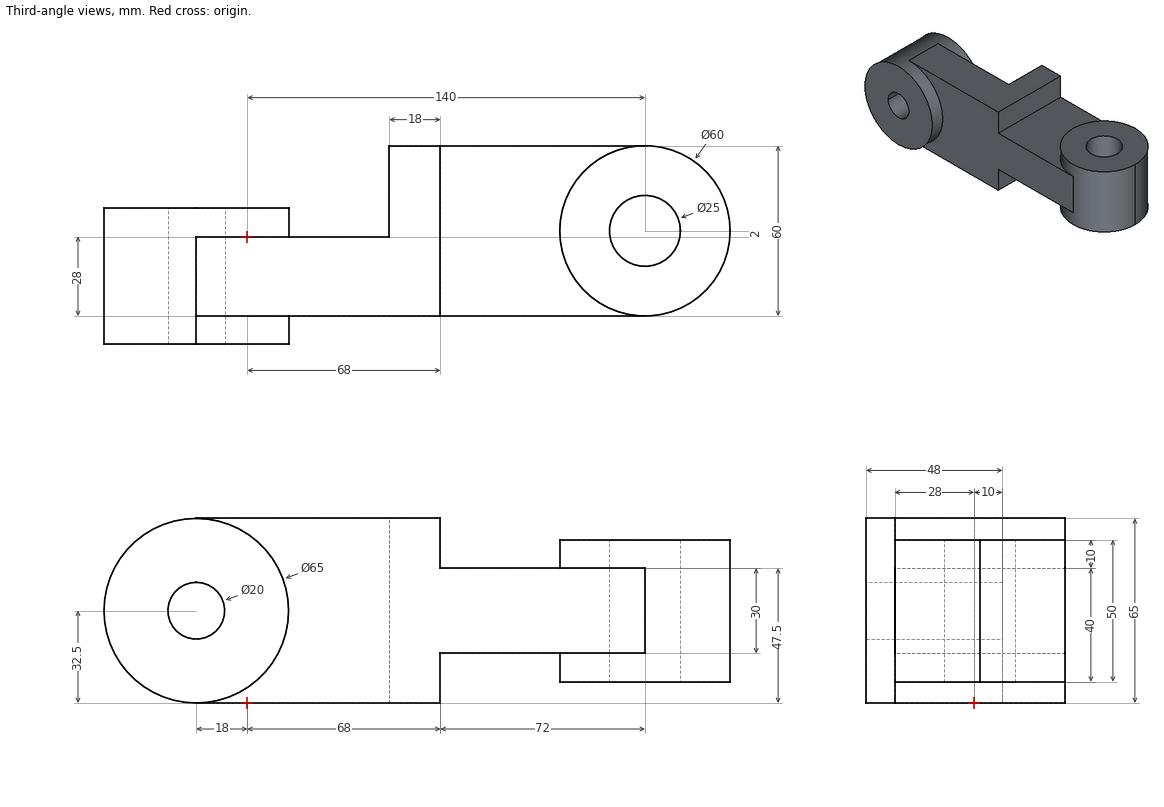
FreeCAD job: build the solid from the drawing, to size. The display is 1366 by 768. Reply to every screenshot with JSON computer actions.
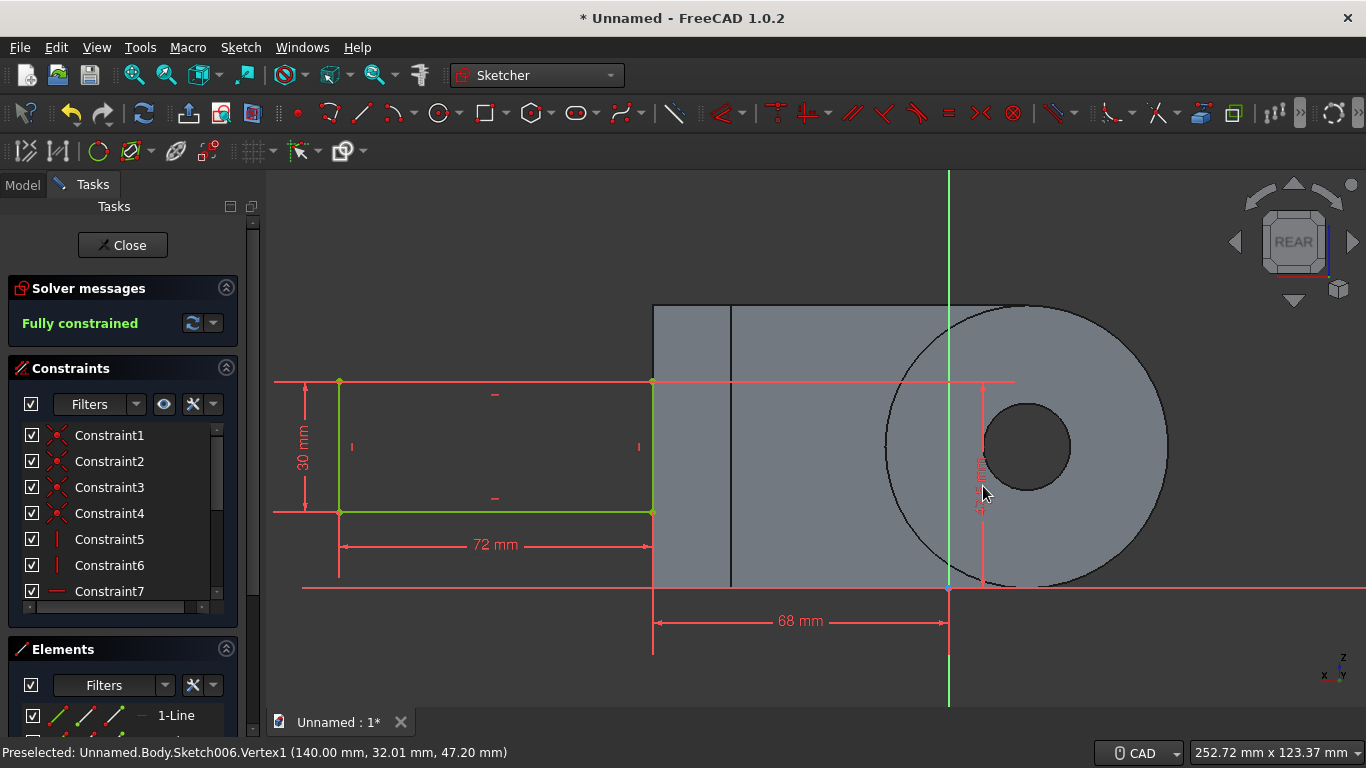
{"action": "left_click", "coordinate": [123, 245]}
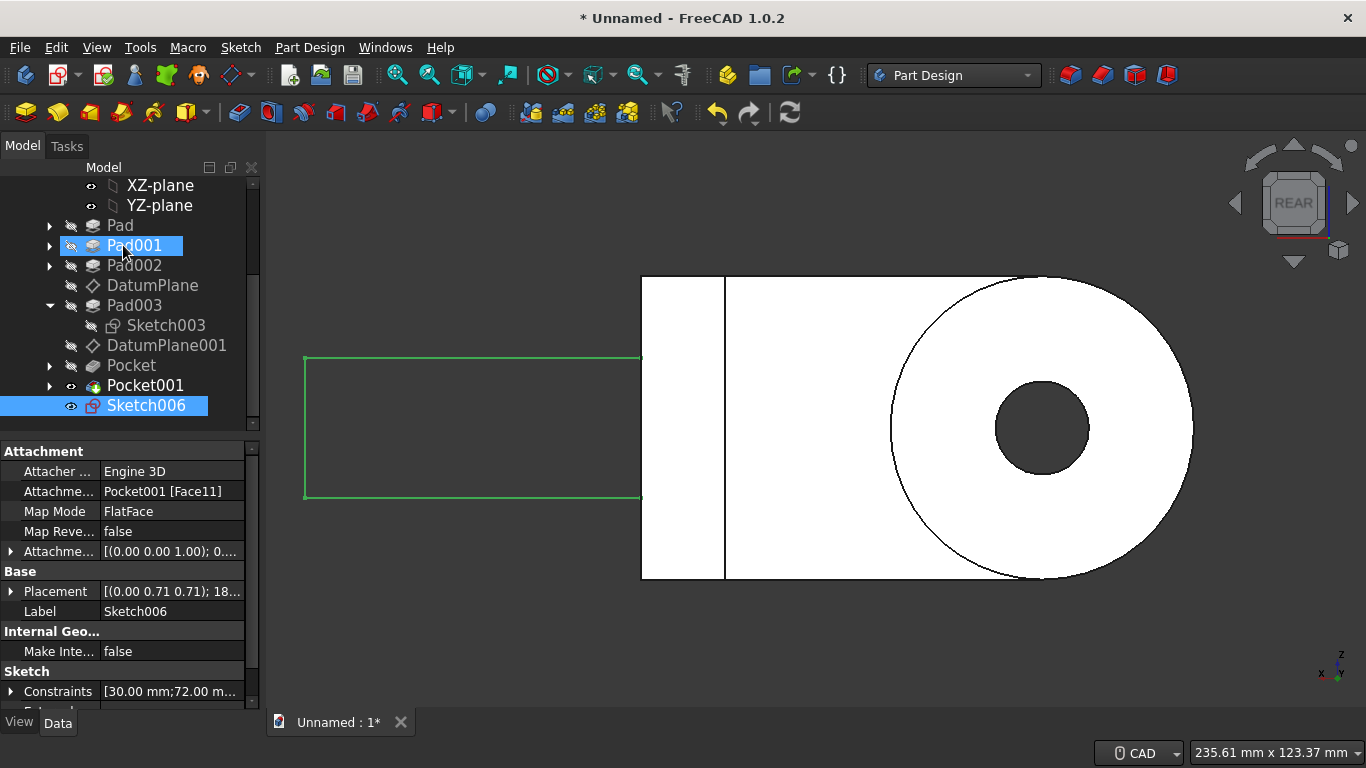
{"action": "left_click", "coordinate": [26, 112]}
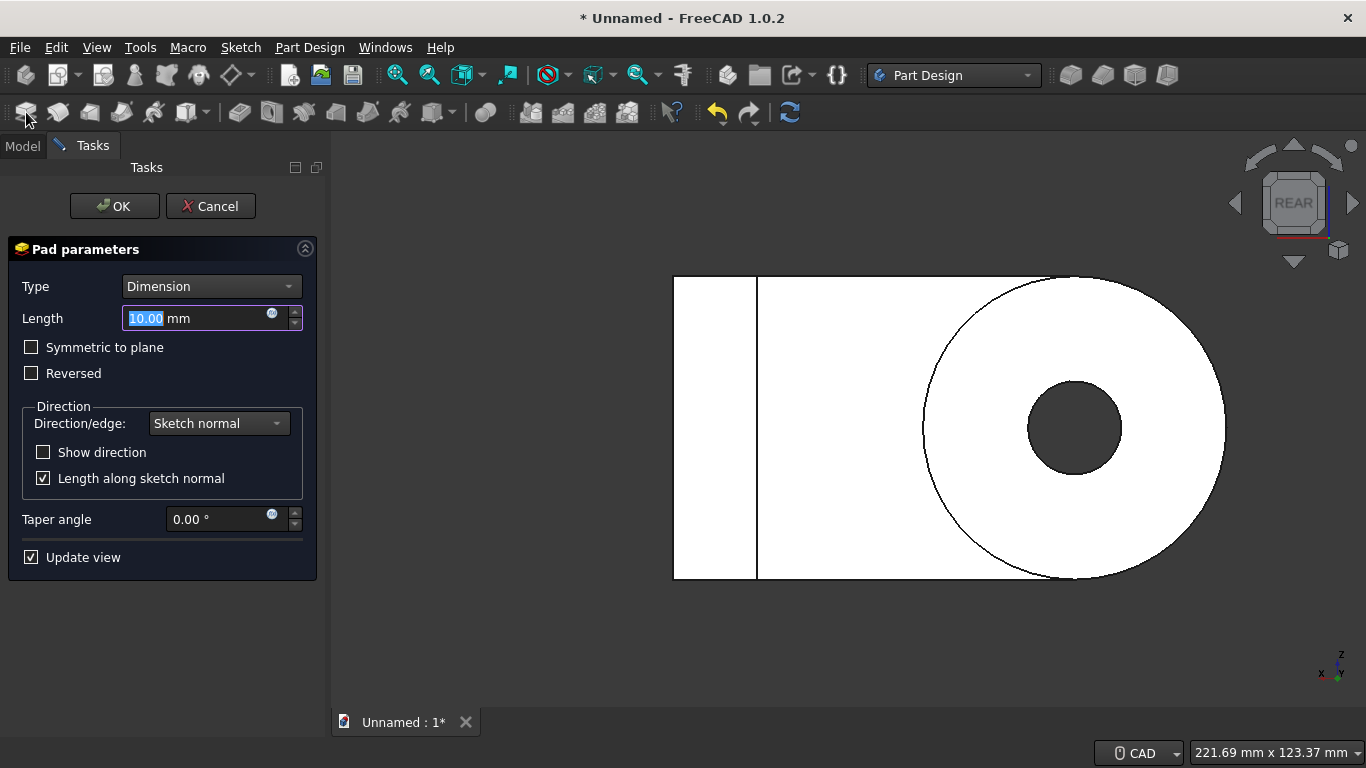
{"action": "type", "text": "60"}
{"action": "key", "text": "Tab"}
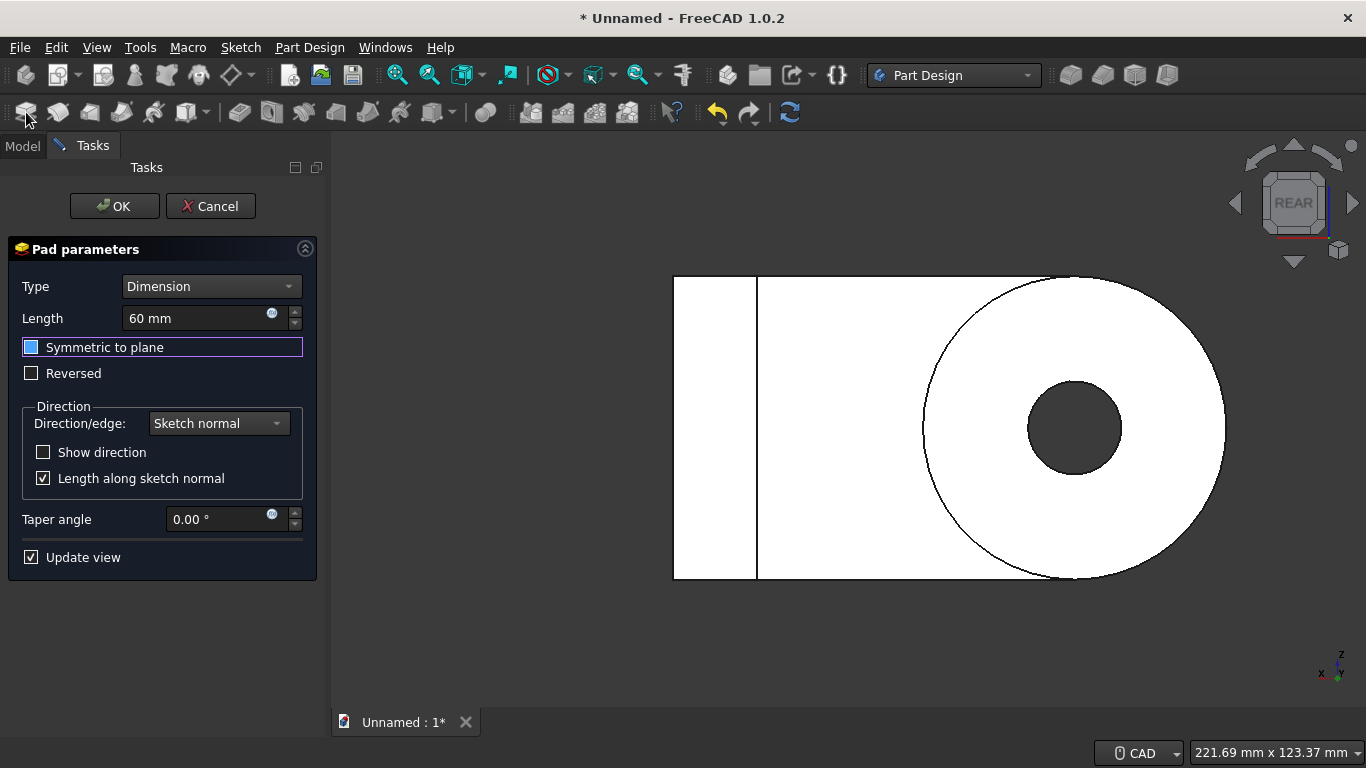
{"action": "left_click", "coordinate": [30, 373]}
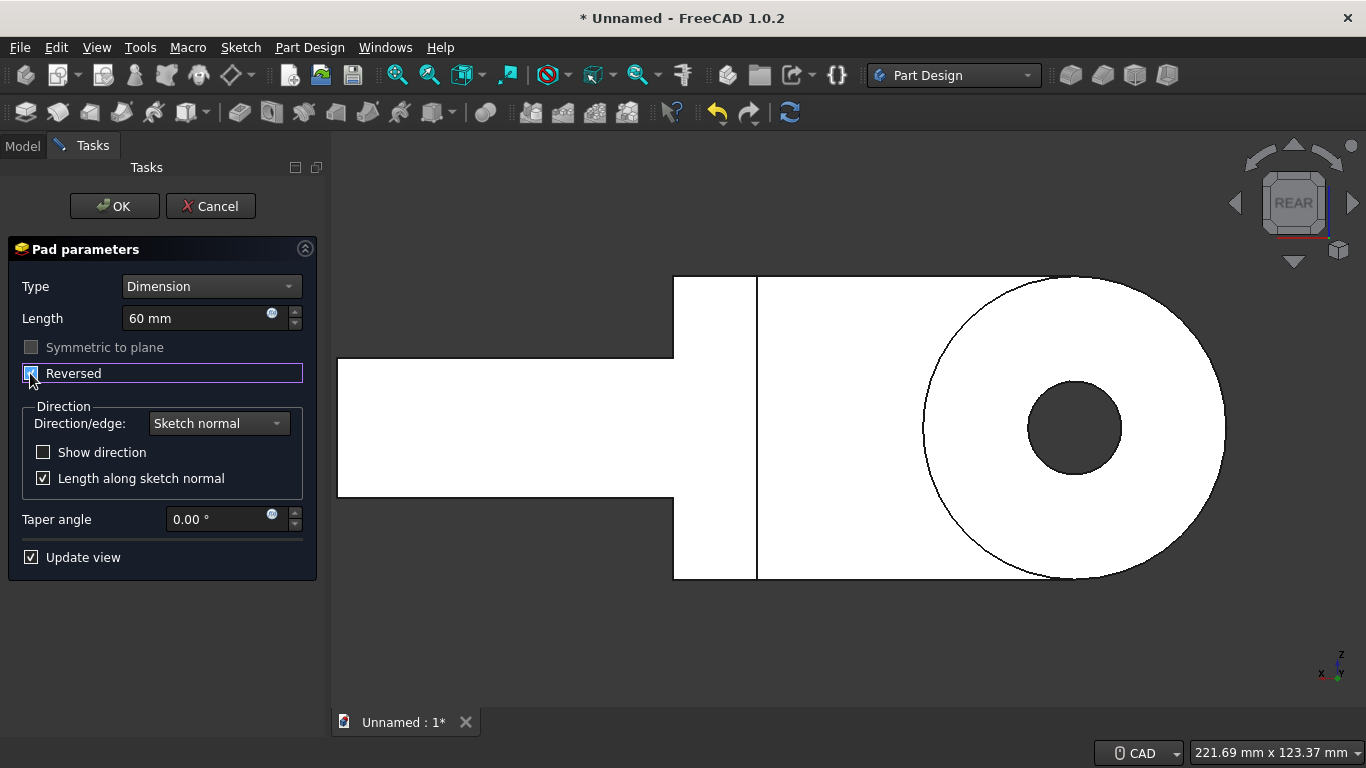
{"action": "left_click", "coordinate": [115, 206]}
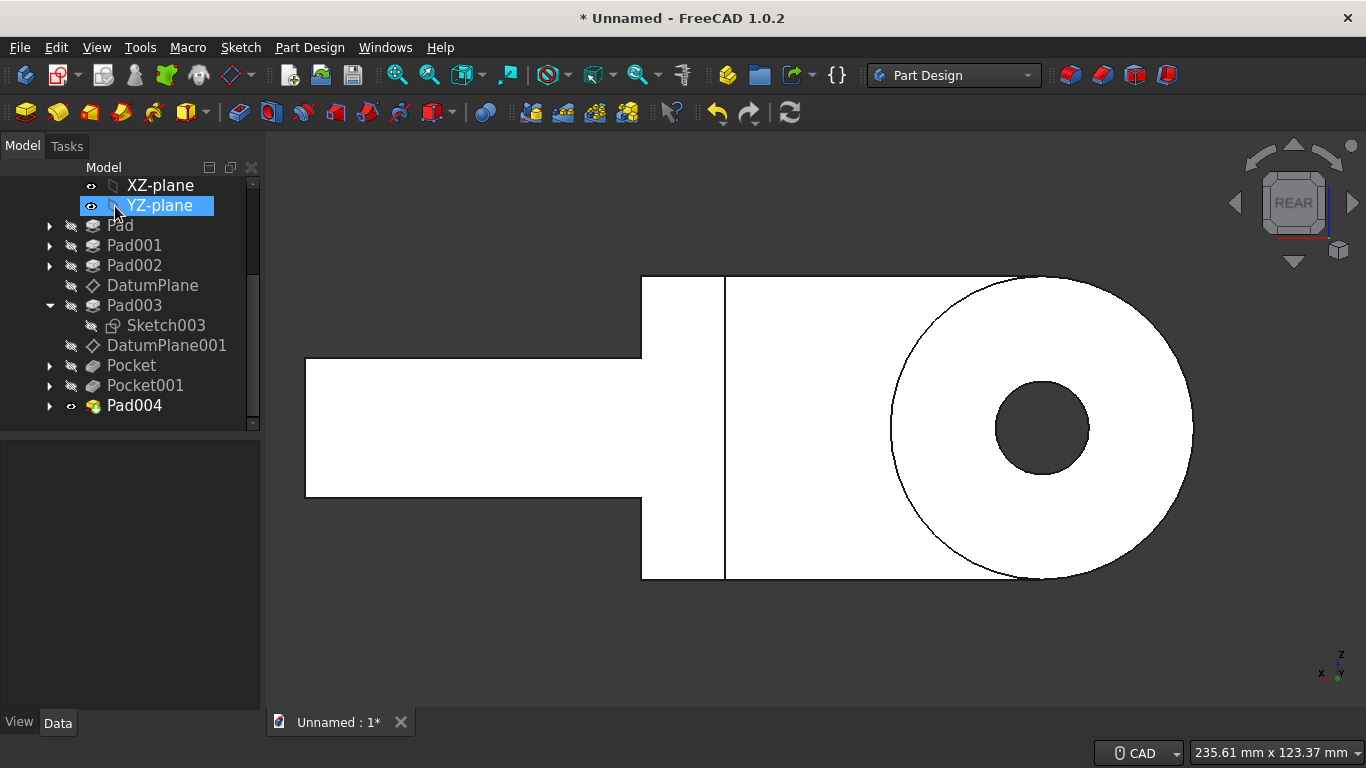
{"action": "key", "text": "0"}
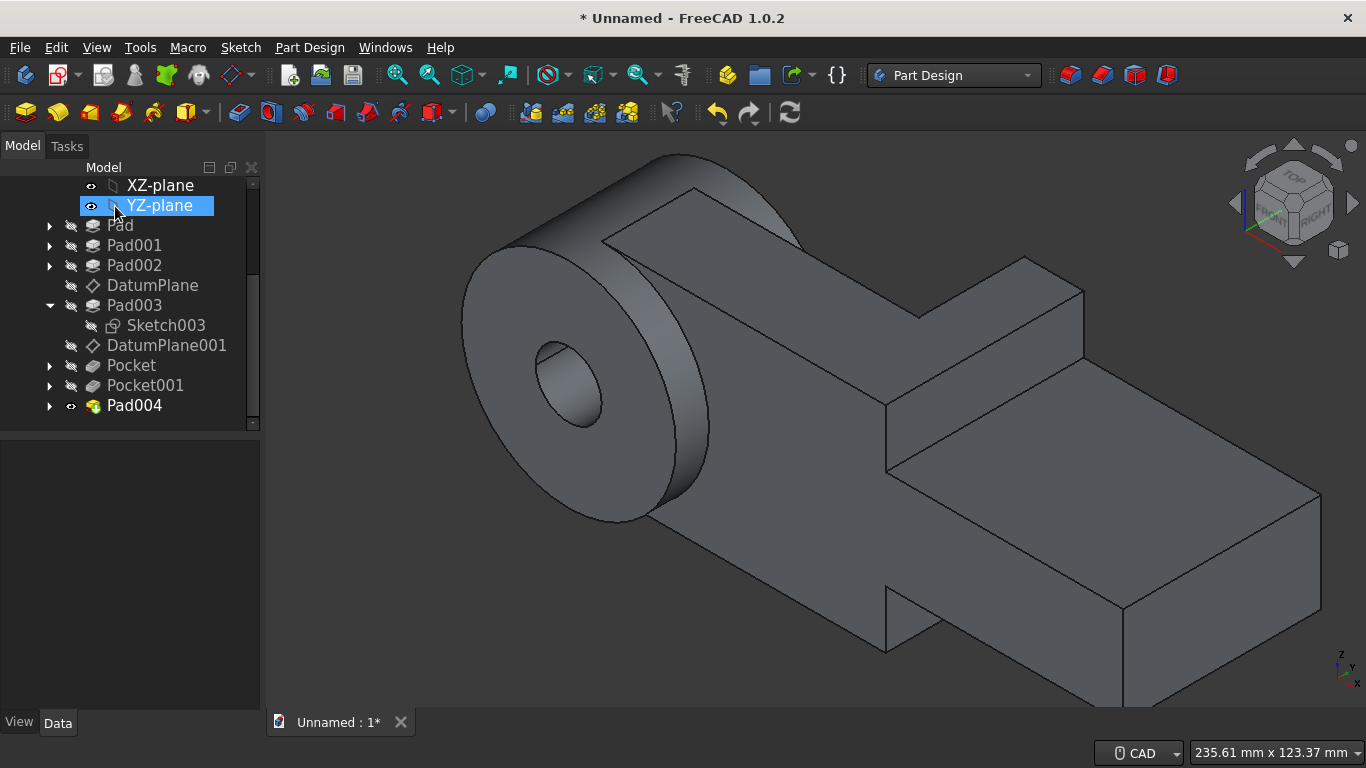
{"action": "left_click", "coordinate": [398, 76]}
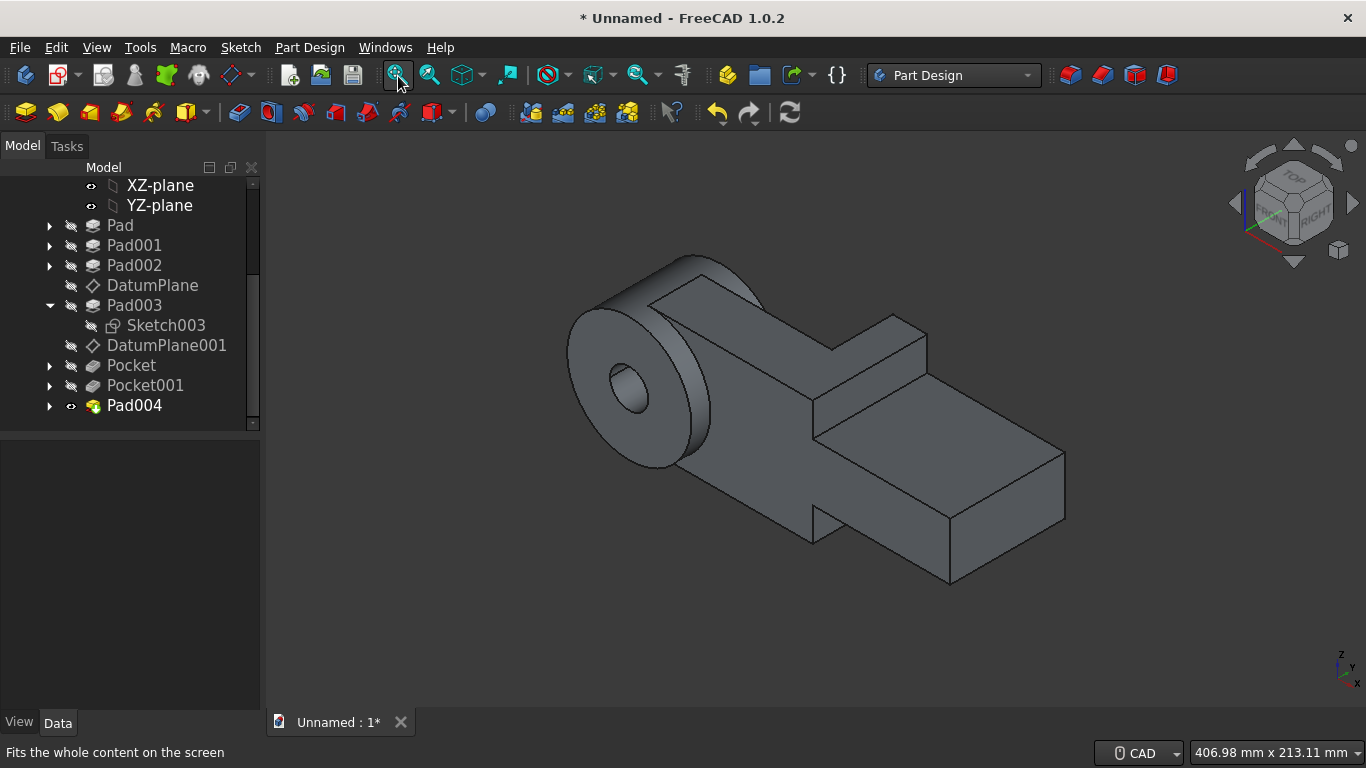
{"action": "left_click", "coordinate": [939, 445]}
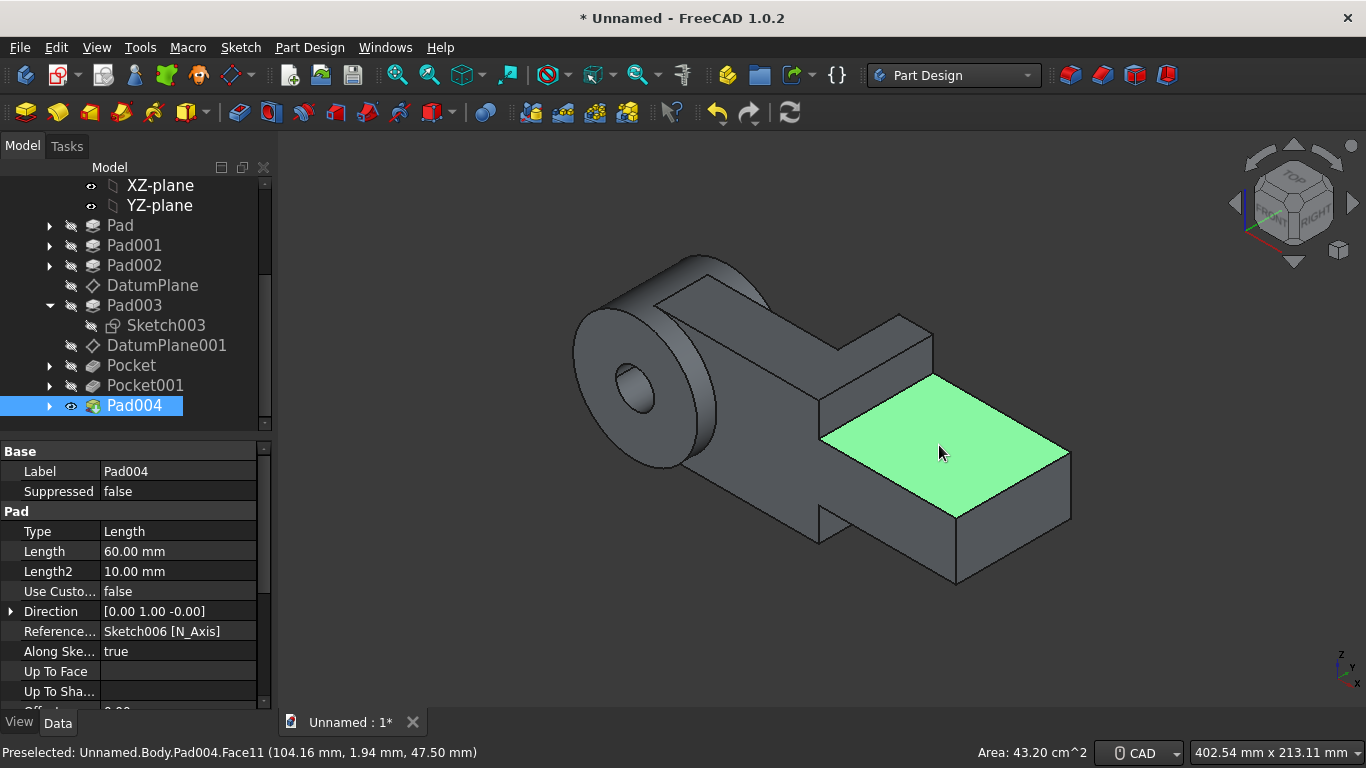
{"action": "left_click", "coordinate": [58, 76]}